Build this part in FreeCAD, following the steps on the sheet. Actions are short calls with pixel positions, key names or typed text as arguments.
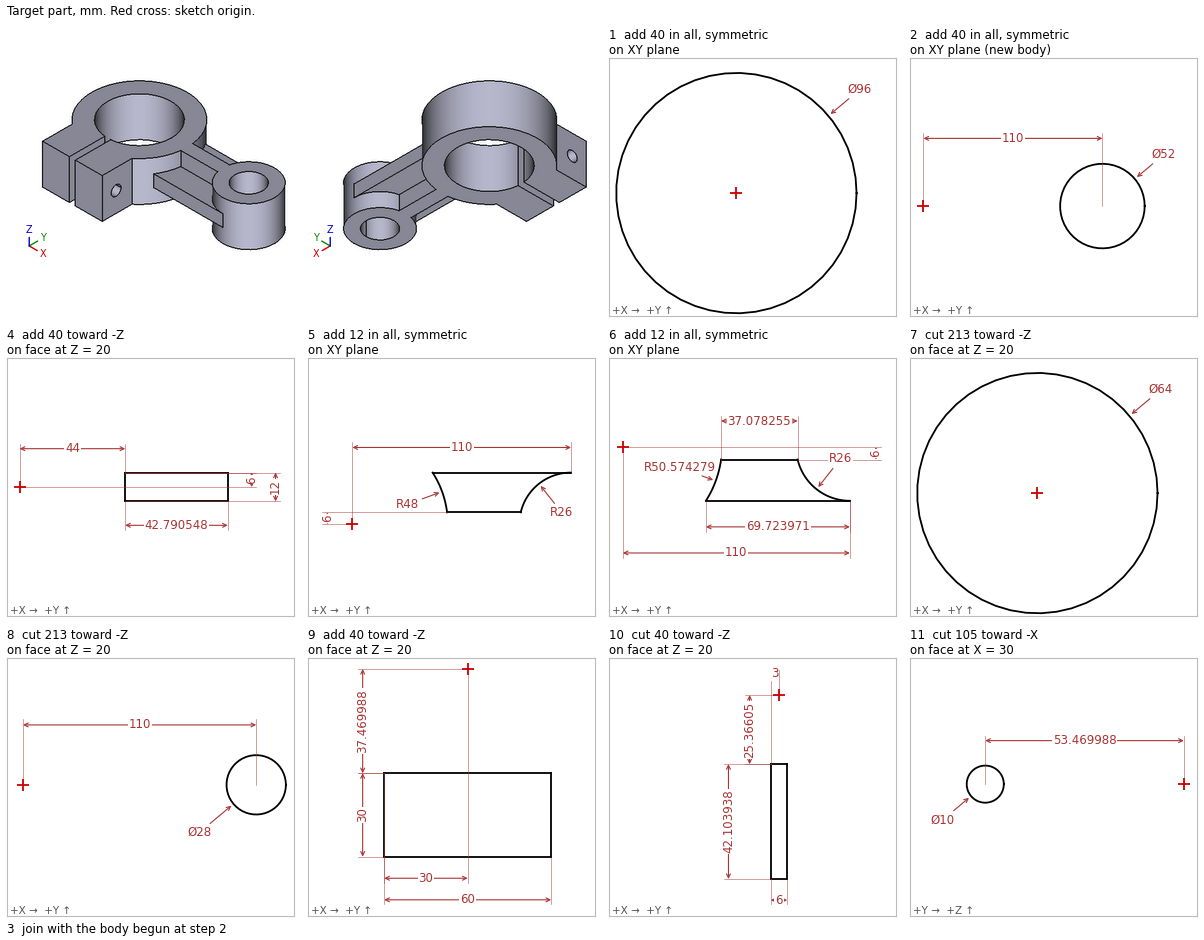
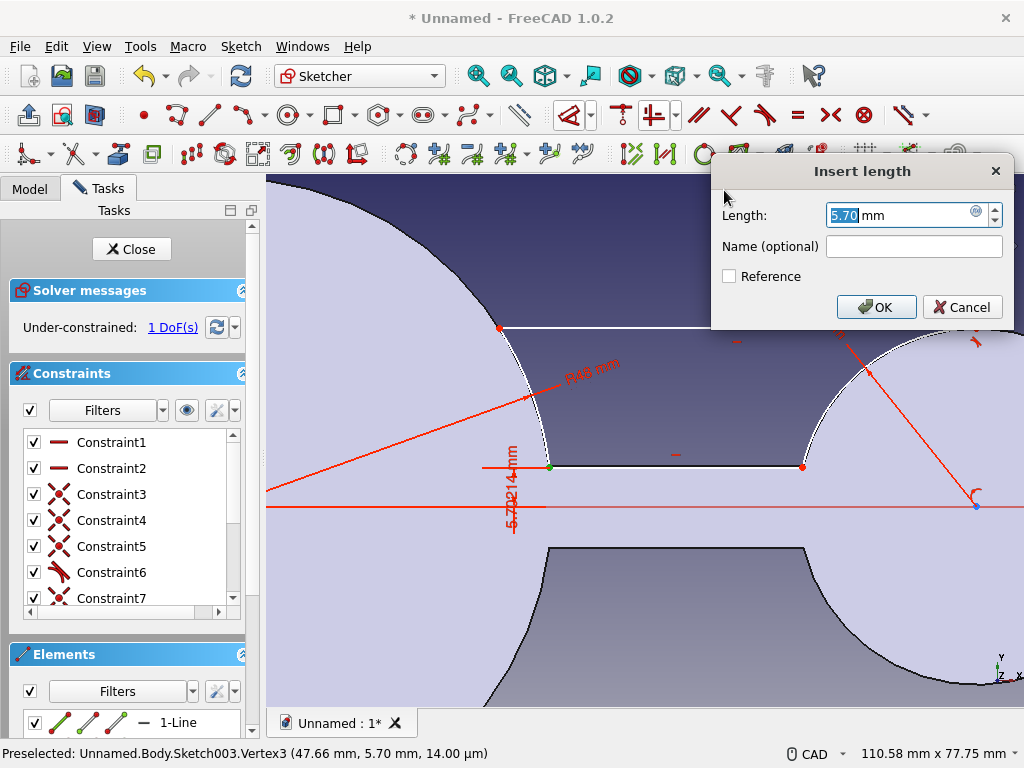
text(6)
key(Return)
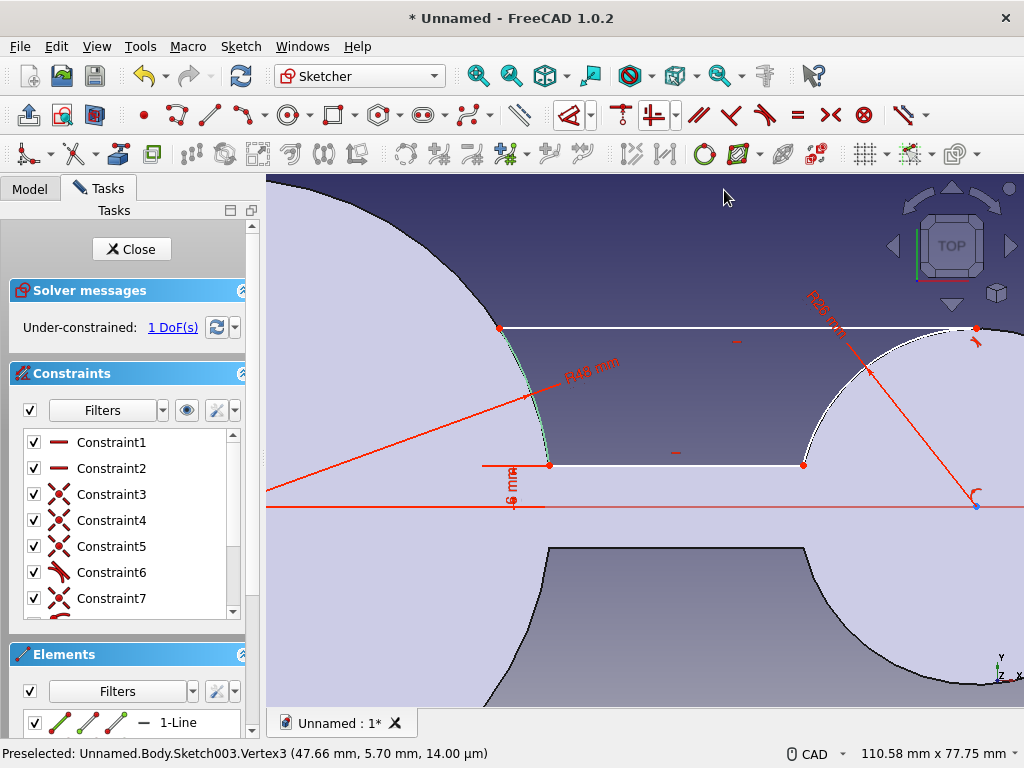
scroll(548, 468, down, 3)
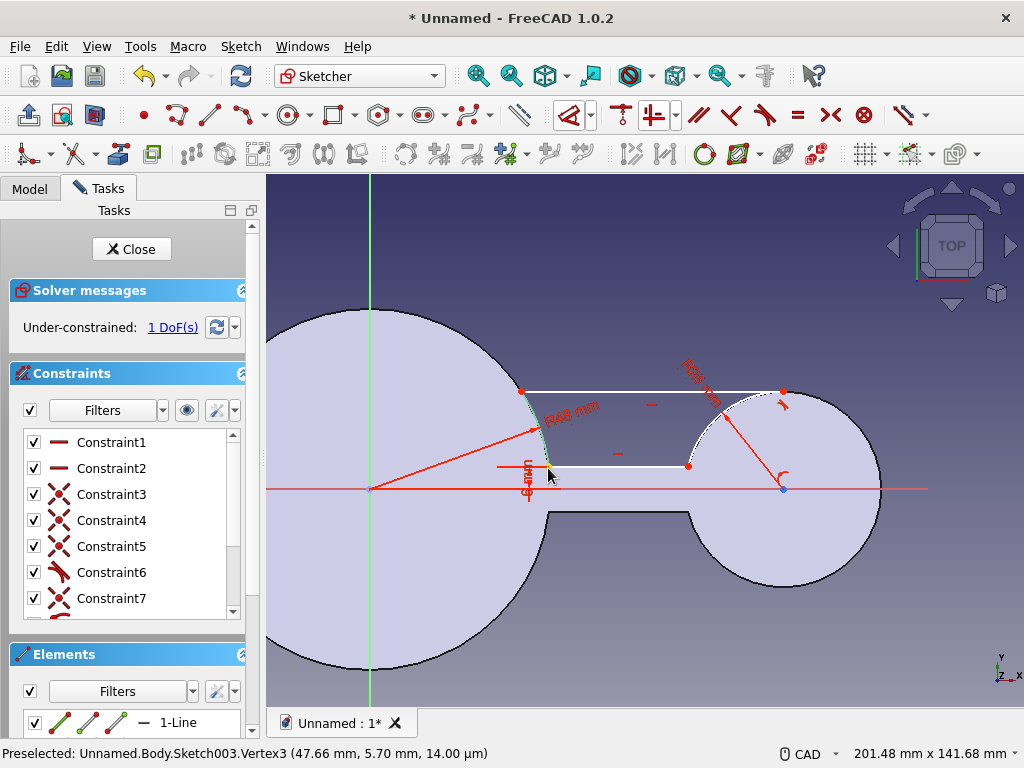
click(783, 392)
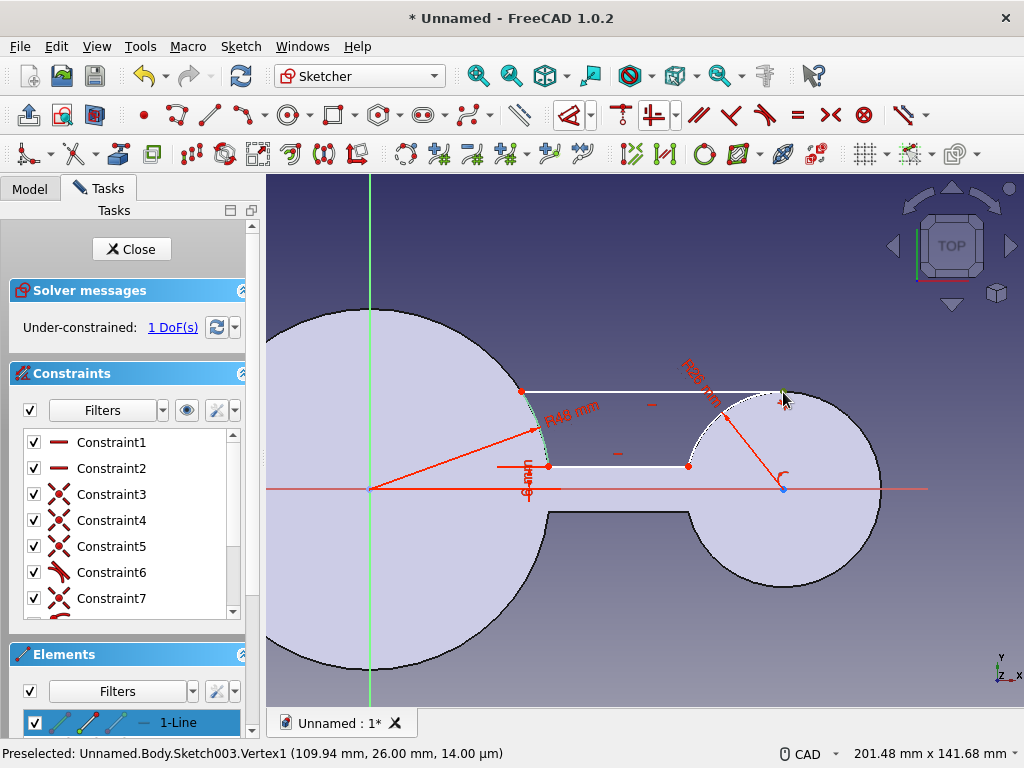
click(590, 116)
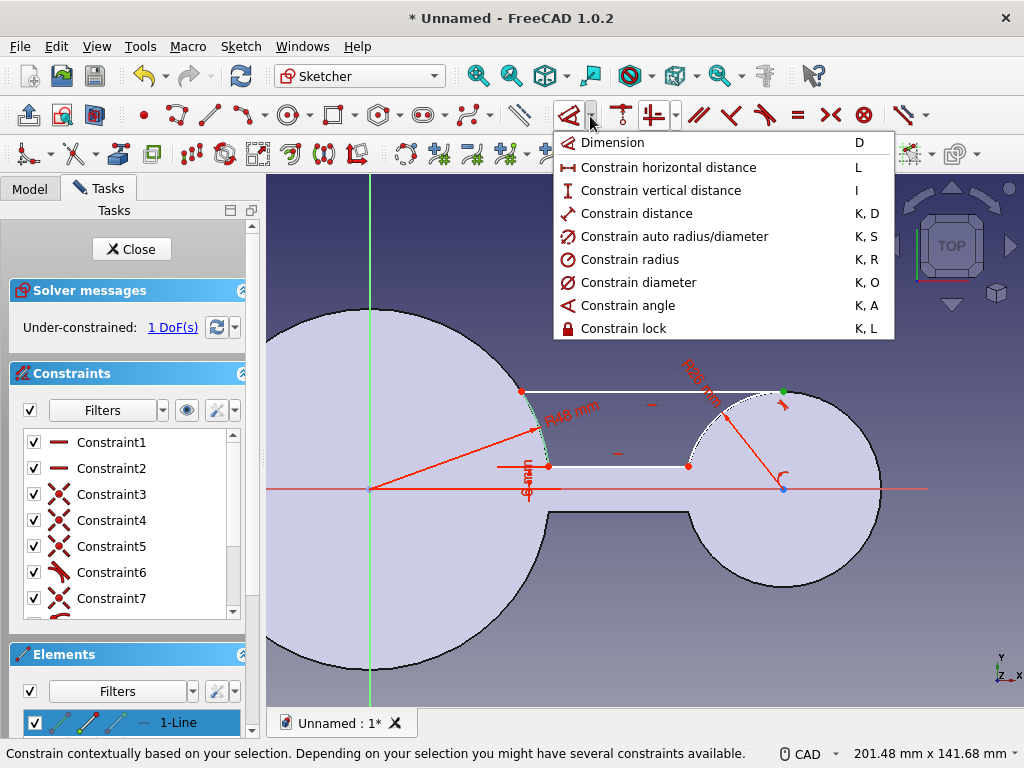
click(724, 168)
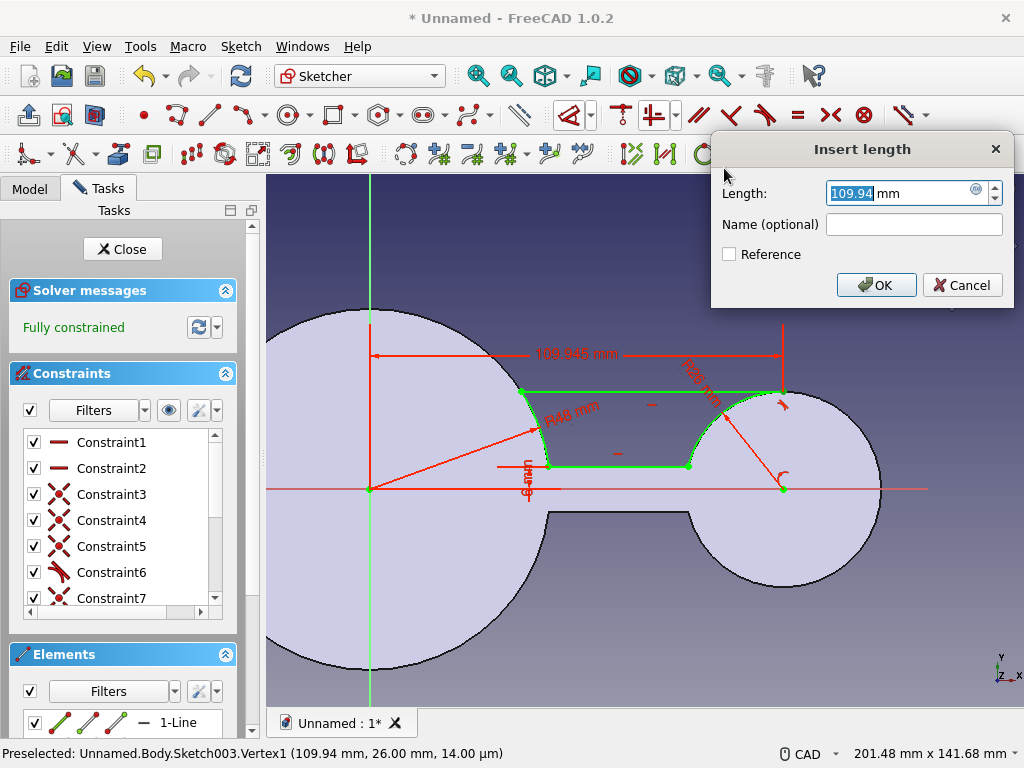
text(110)
key(Return)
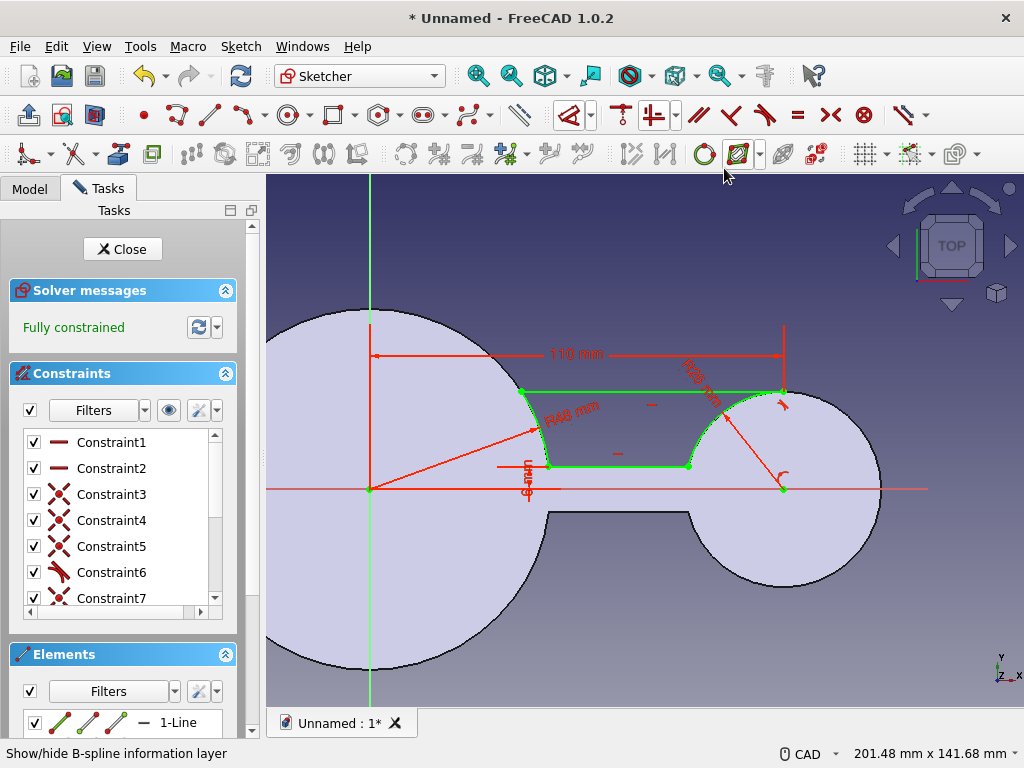
click(123, 249)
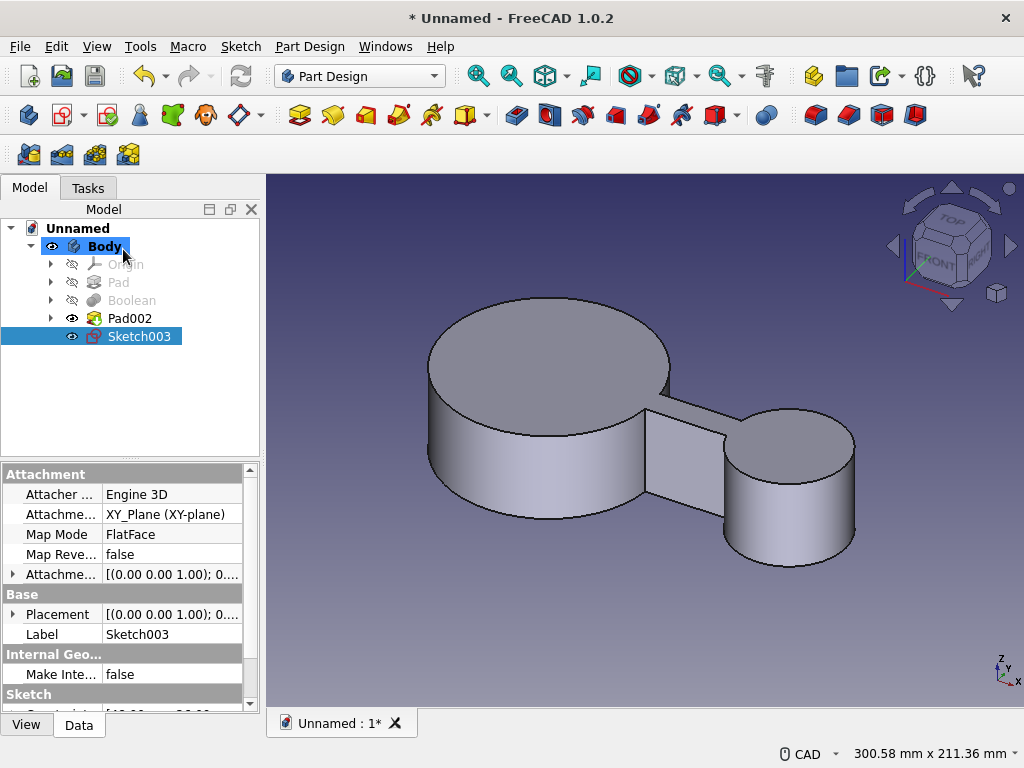
click(300, 116)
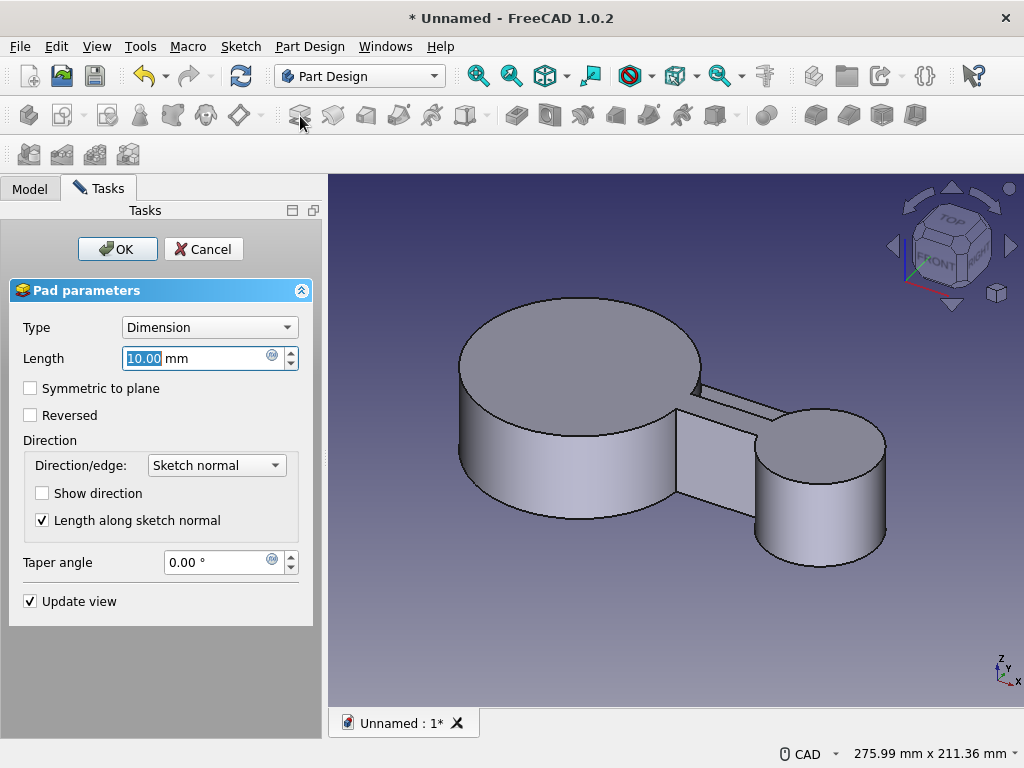
text(12)
key(Tab)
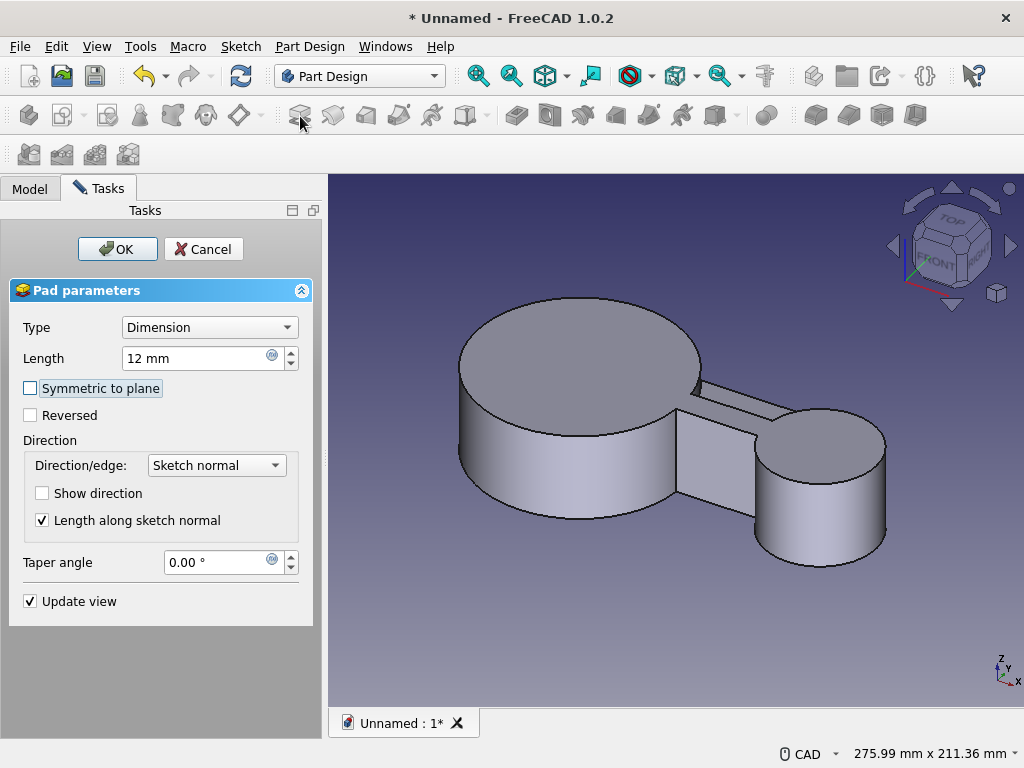
click(31, 388)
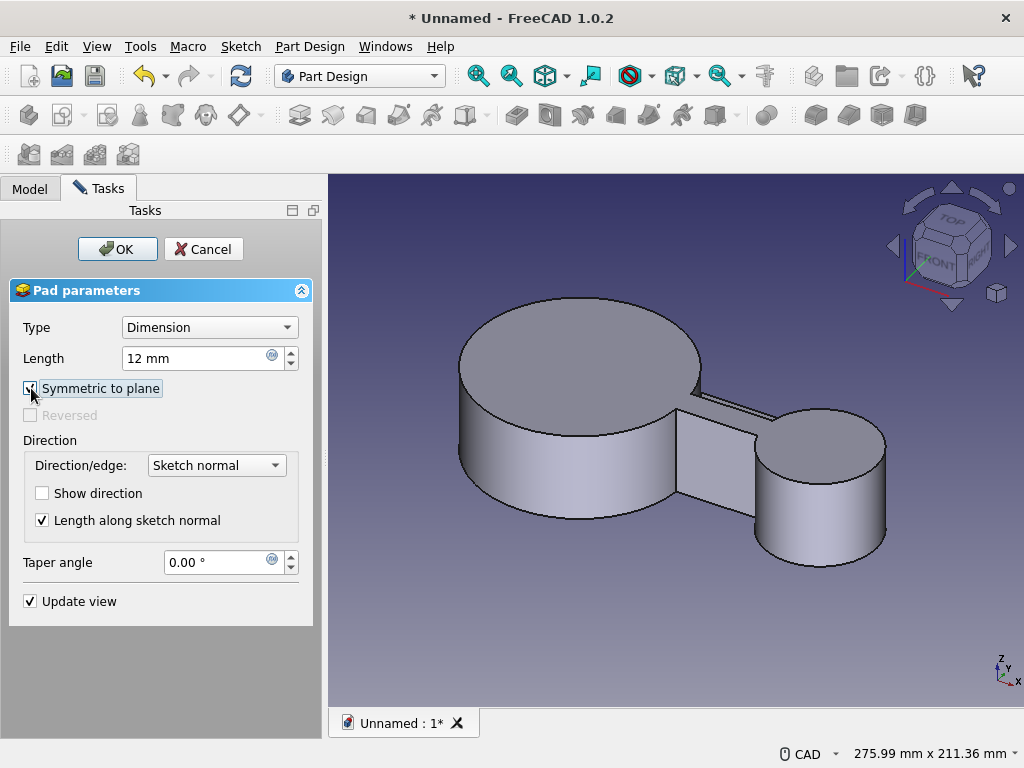
click(118, 249)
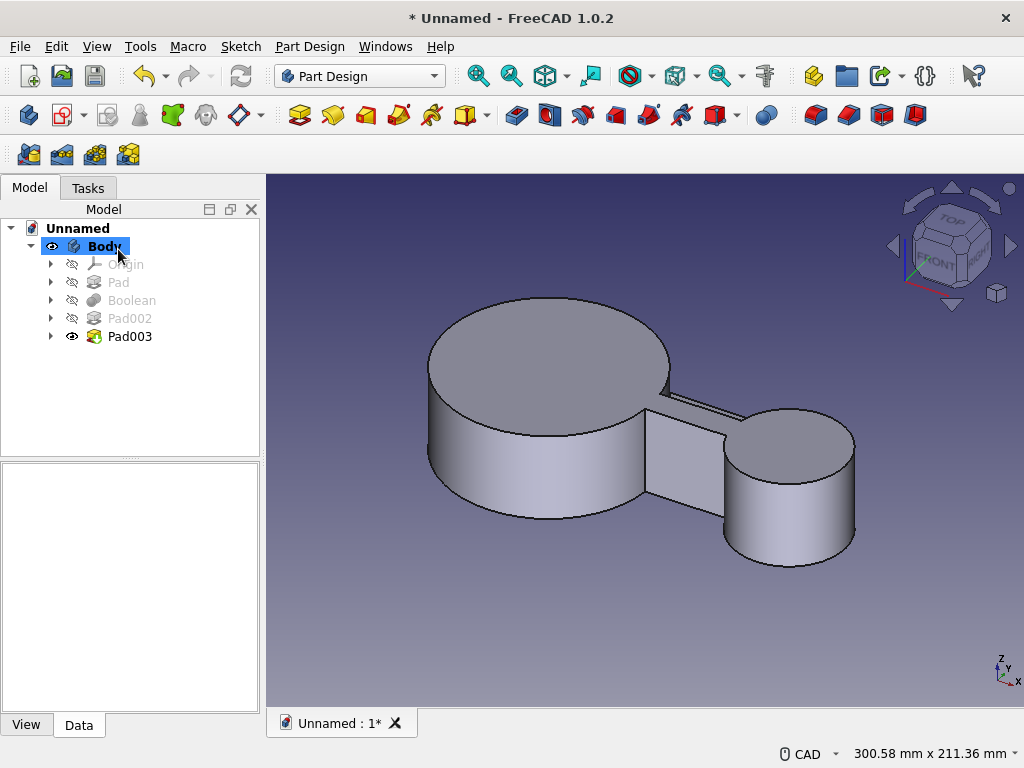
click(62, 116)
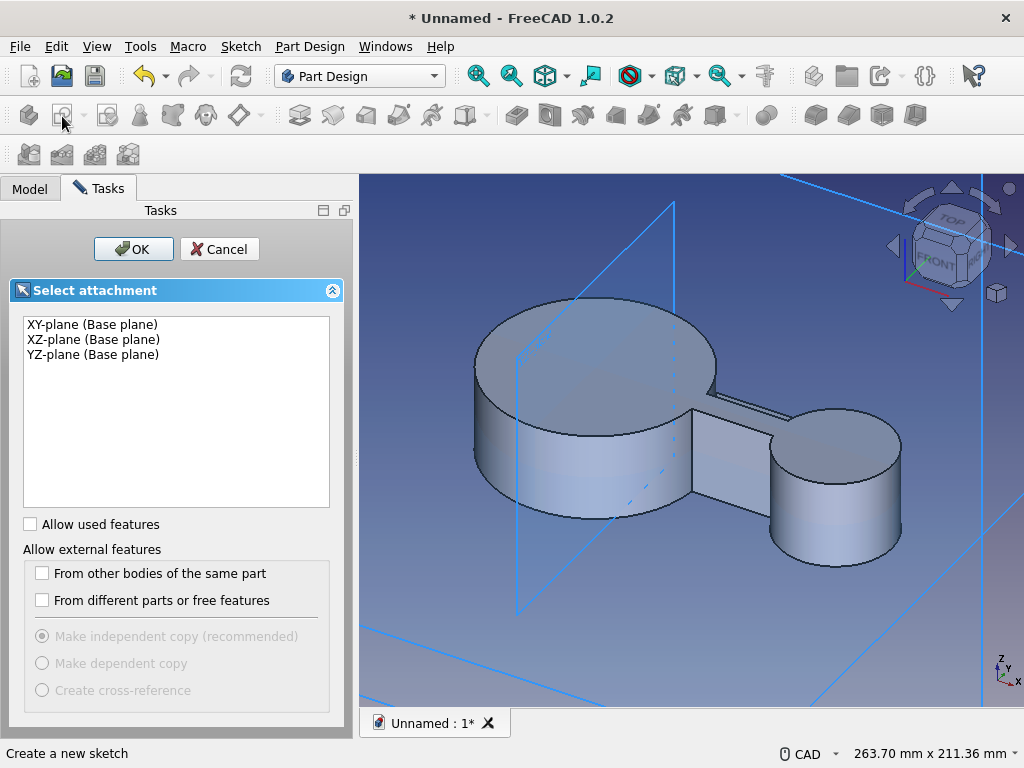
click(84, 324)